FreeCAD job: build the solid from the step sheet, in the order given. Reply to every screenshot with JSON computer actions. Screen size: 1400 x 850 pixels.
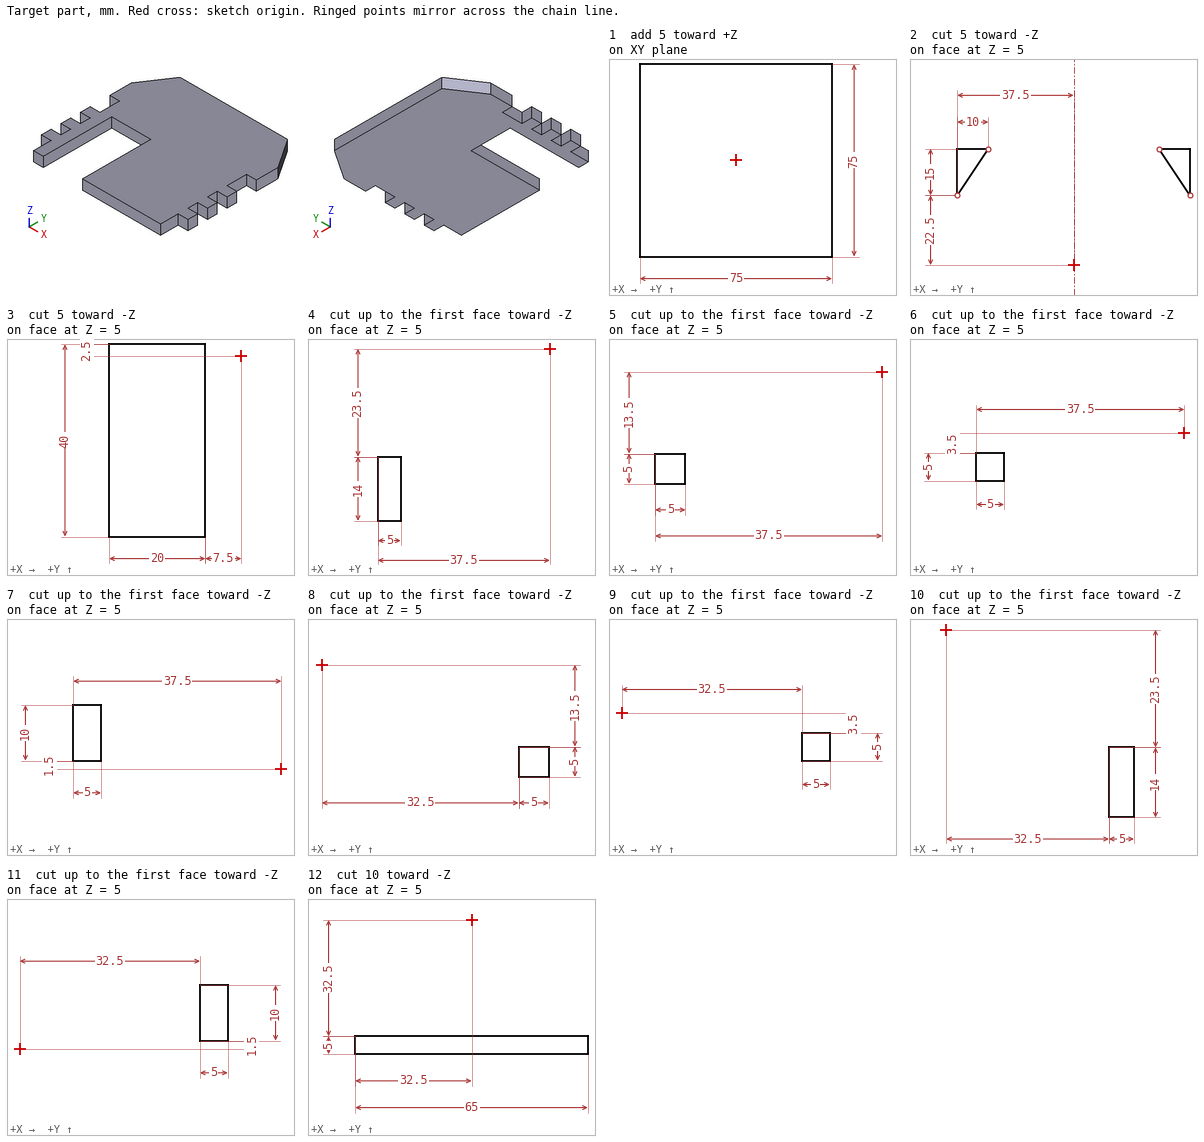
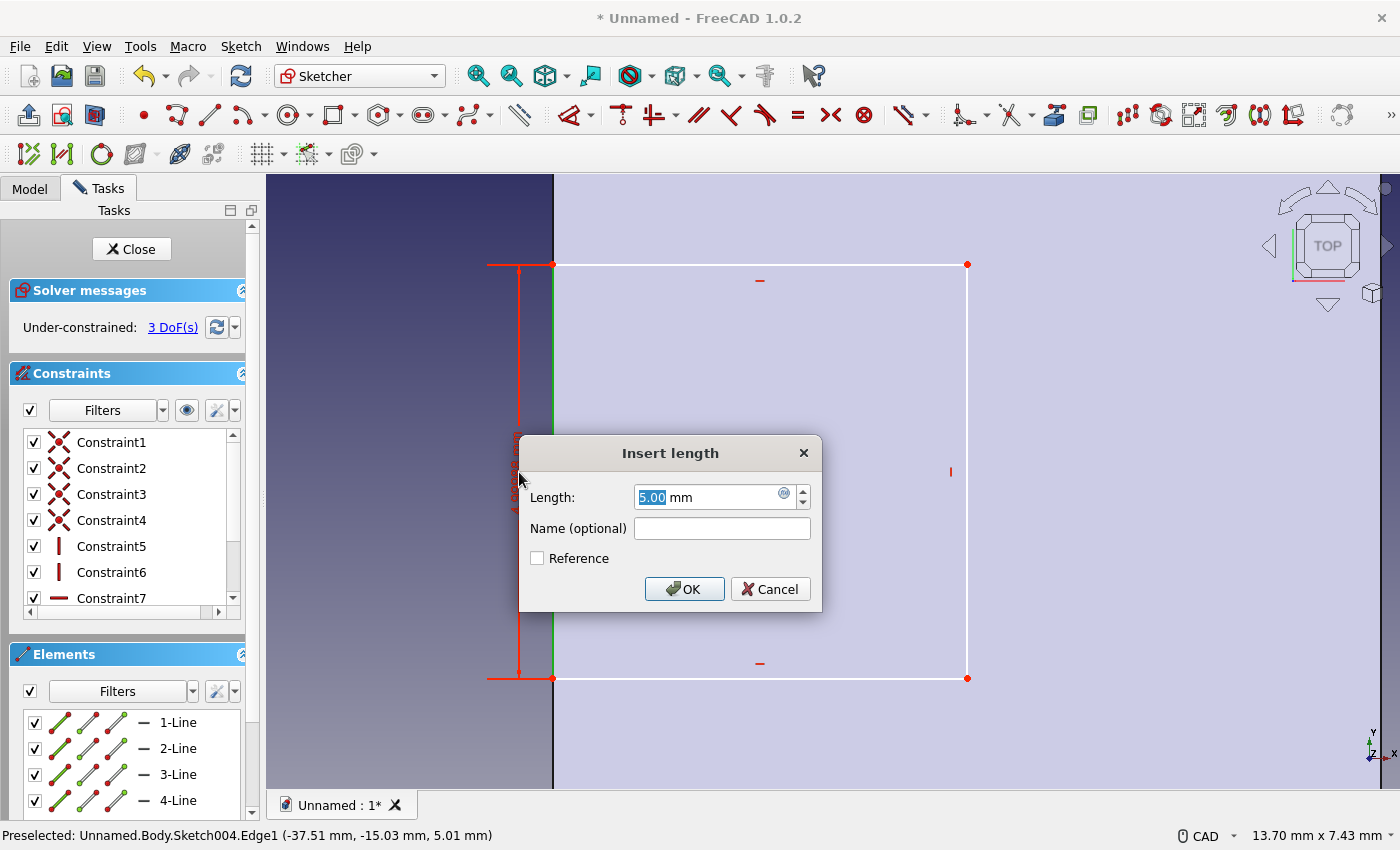
{"action": "type", "text": "5"}
{"action": "key", "text": "Return"}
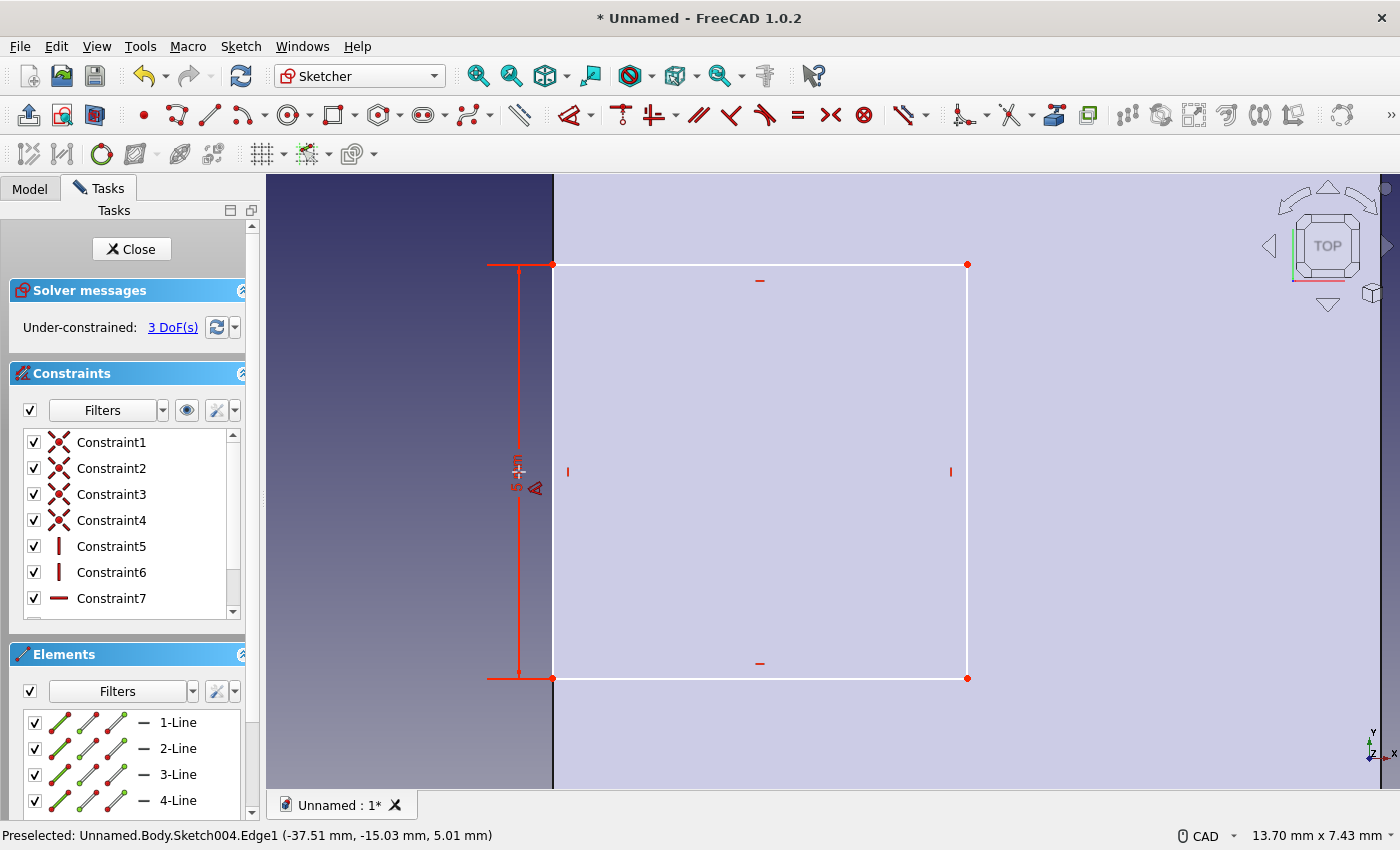
{"action": "left_click", "coordinate": [677, 679]}
{"action": "left_click", "coordinate": [760, 713]}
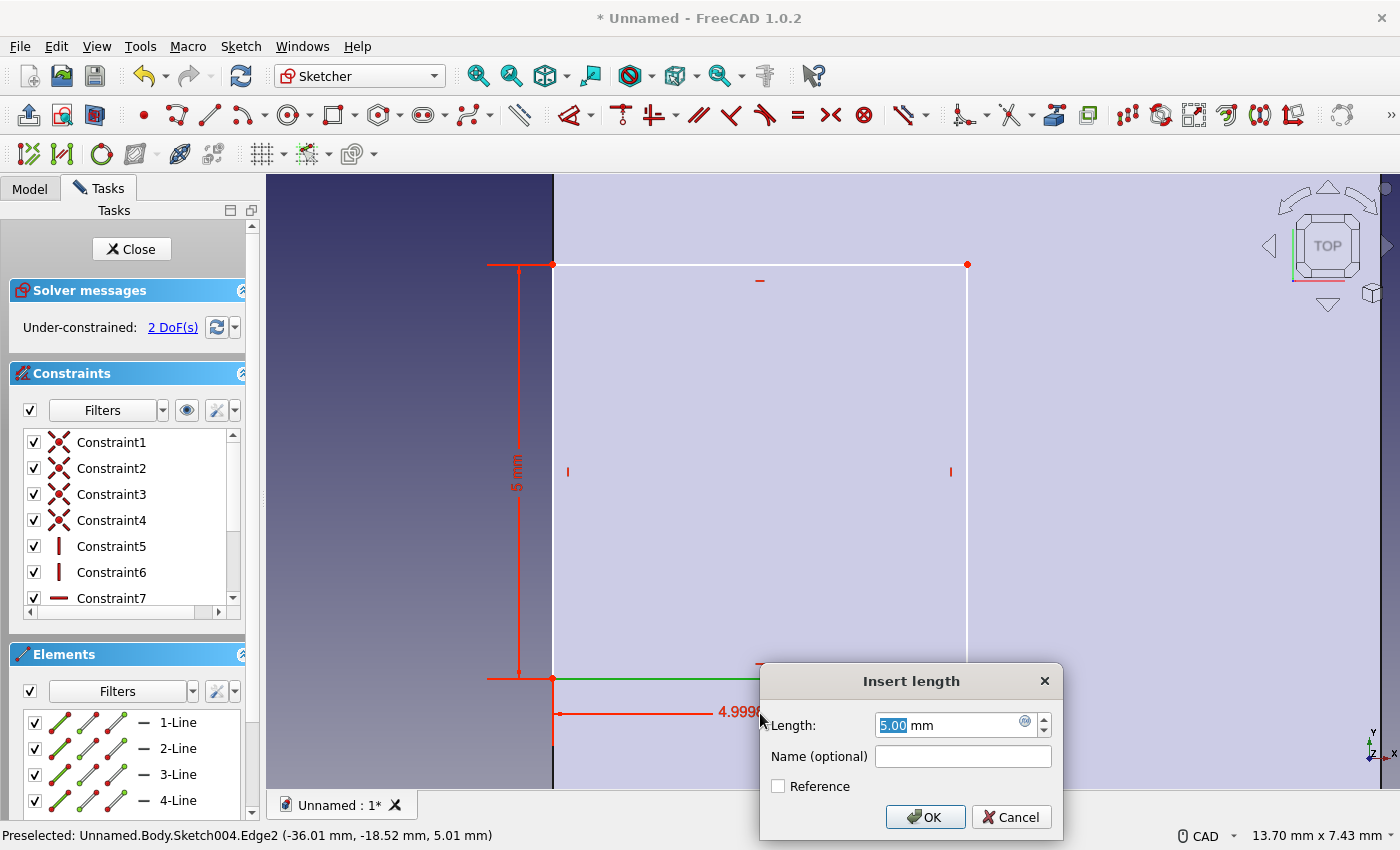
{"action": "type", "text": "5"}
{"action": "key", "text": "Return"}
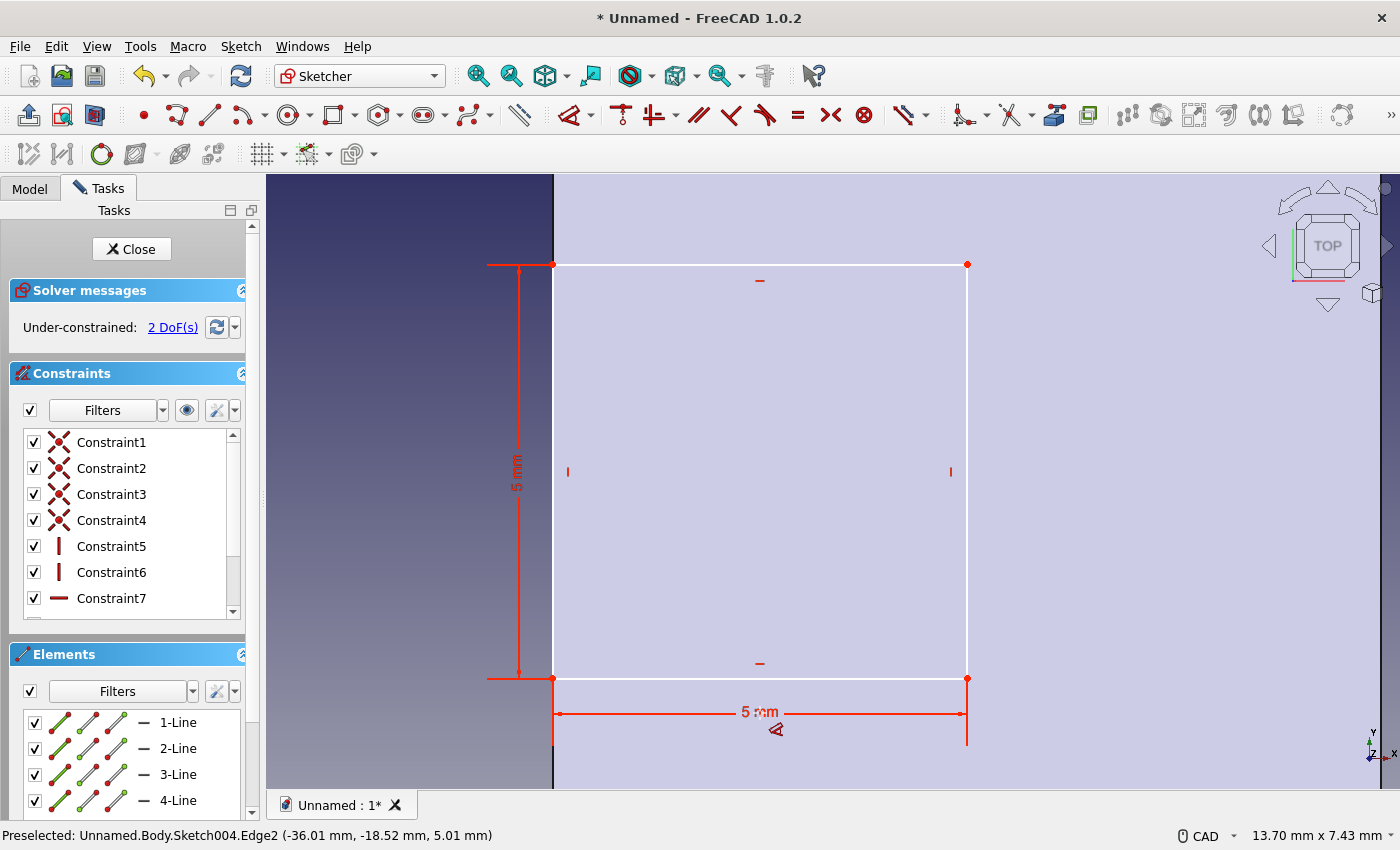
{"action": "left_click", "coordinate": [553, 265]}
{"action": "left_click", "coordinate": [894, 299]}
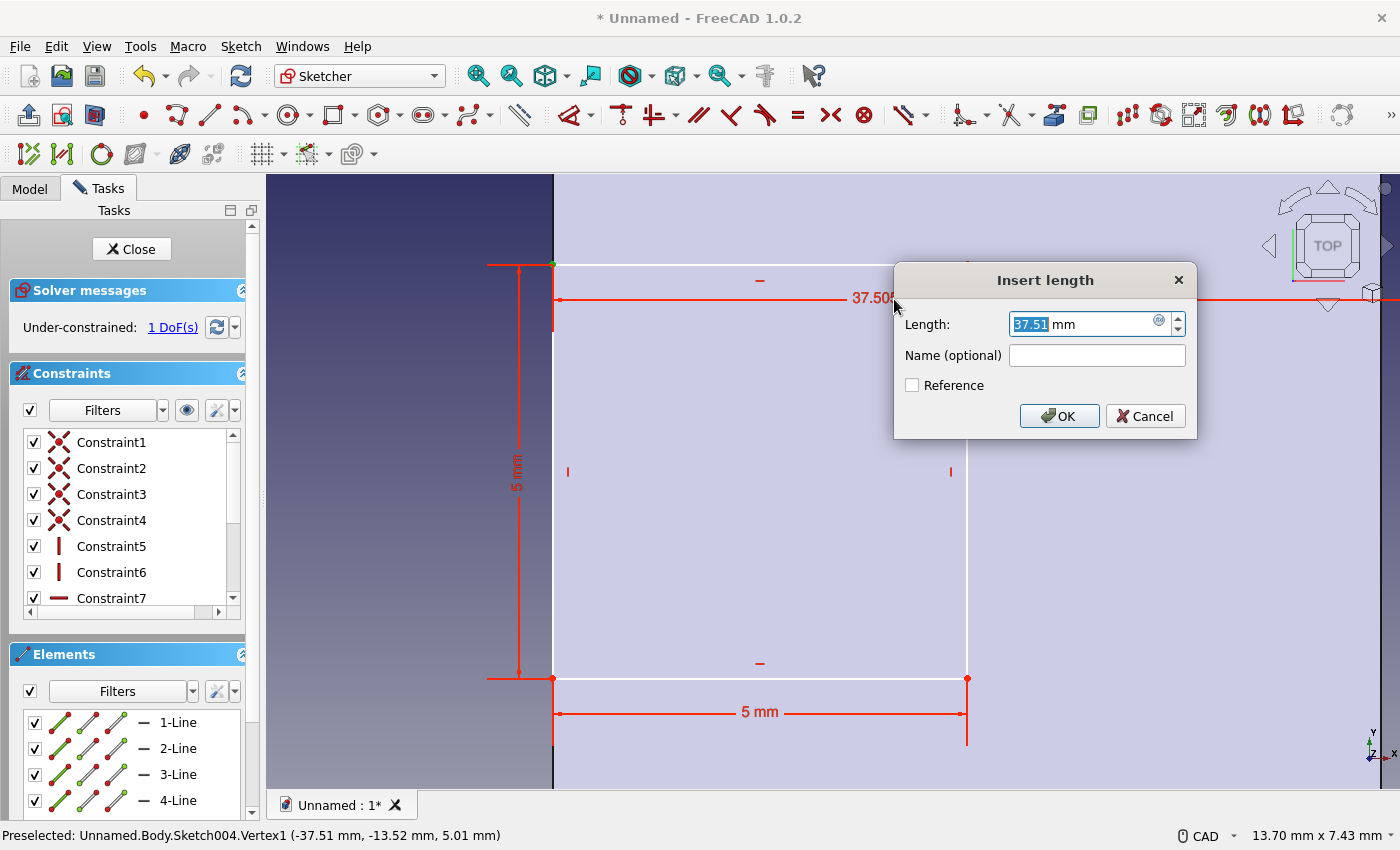
{"action": "type", "text": "37.5"}
{"action": "key", "text": "Return"}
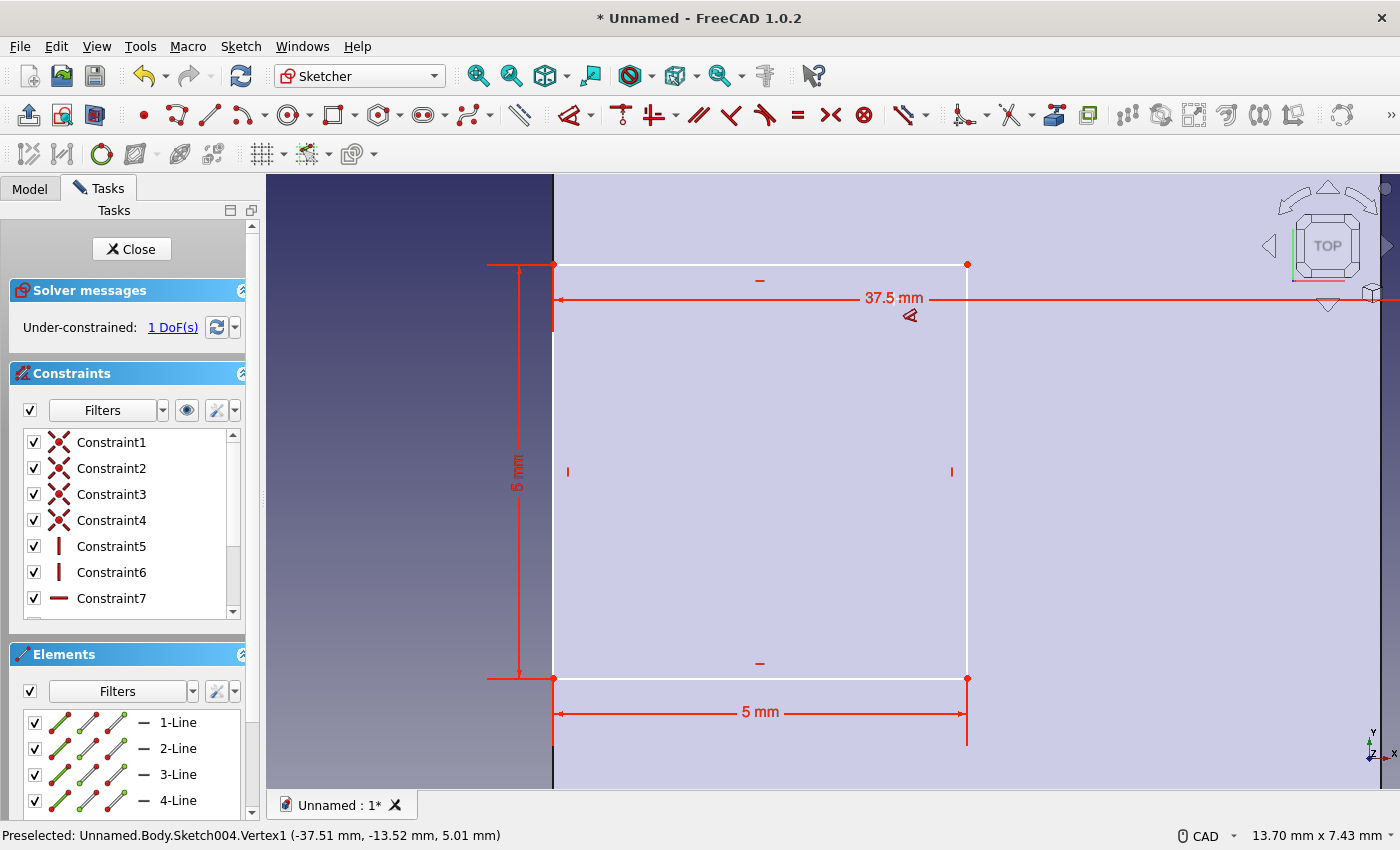
{"action": "left_click", "coordinate": [553, 265]}
{"action": "left_click", "coordinate": [519, 233]}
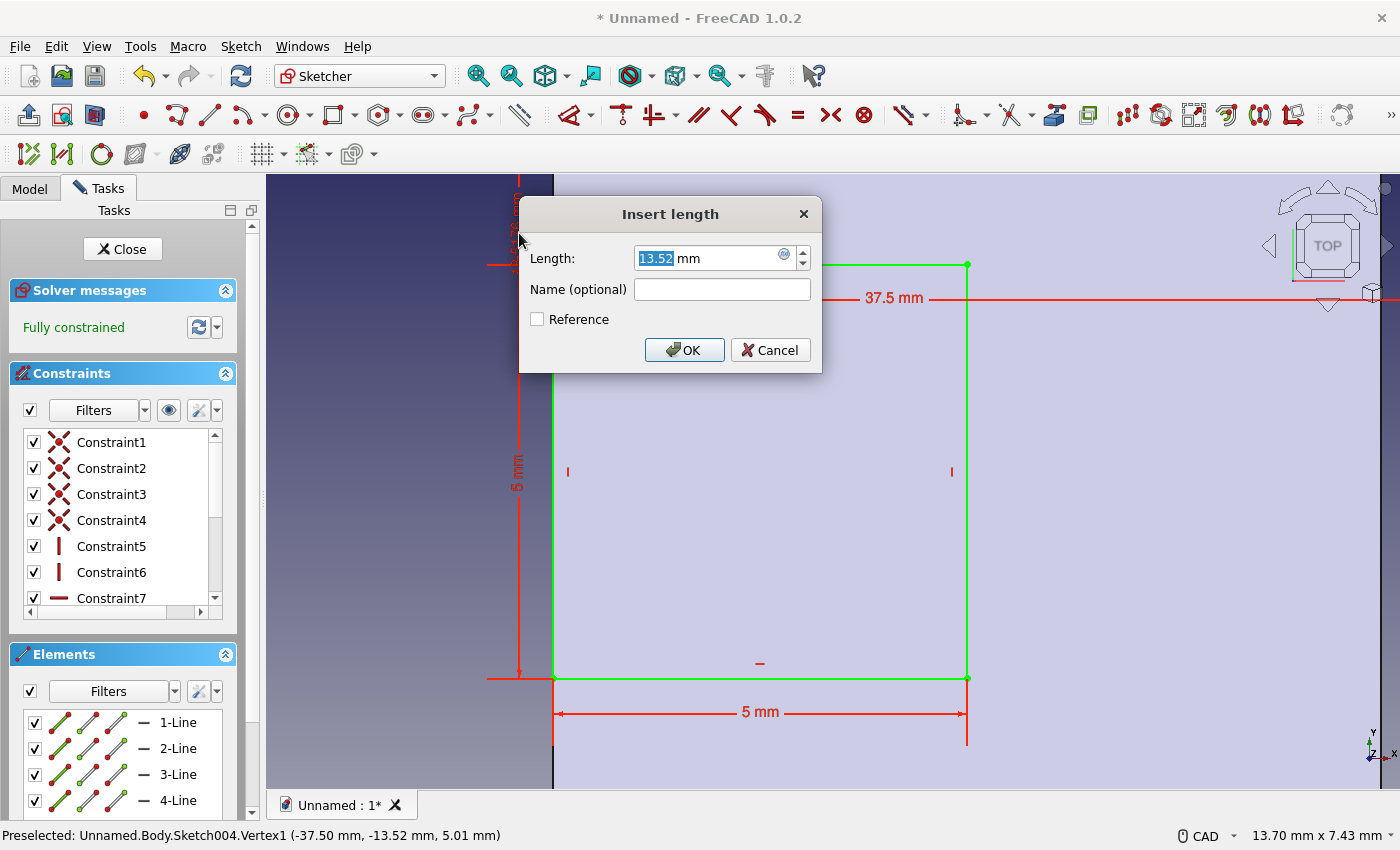
{"action": "type", "text": "13.5"}
{"action": "key", "text": "Return"}
{"action": "key", "text": "Escape"}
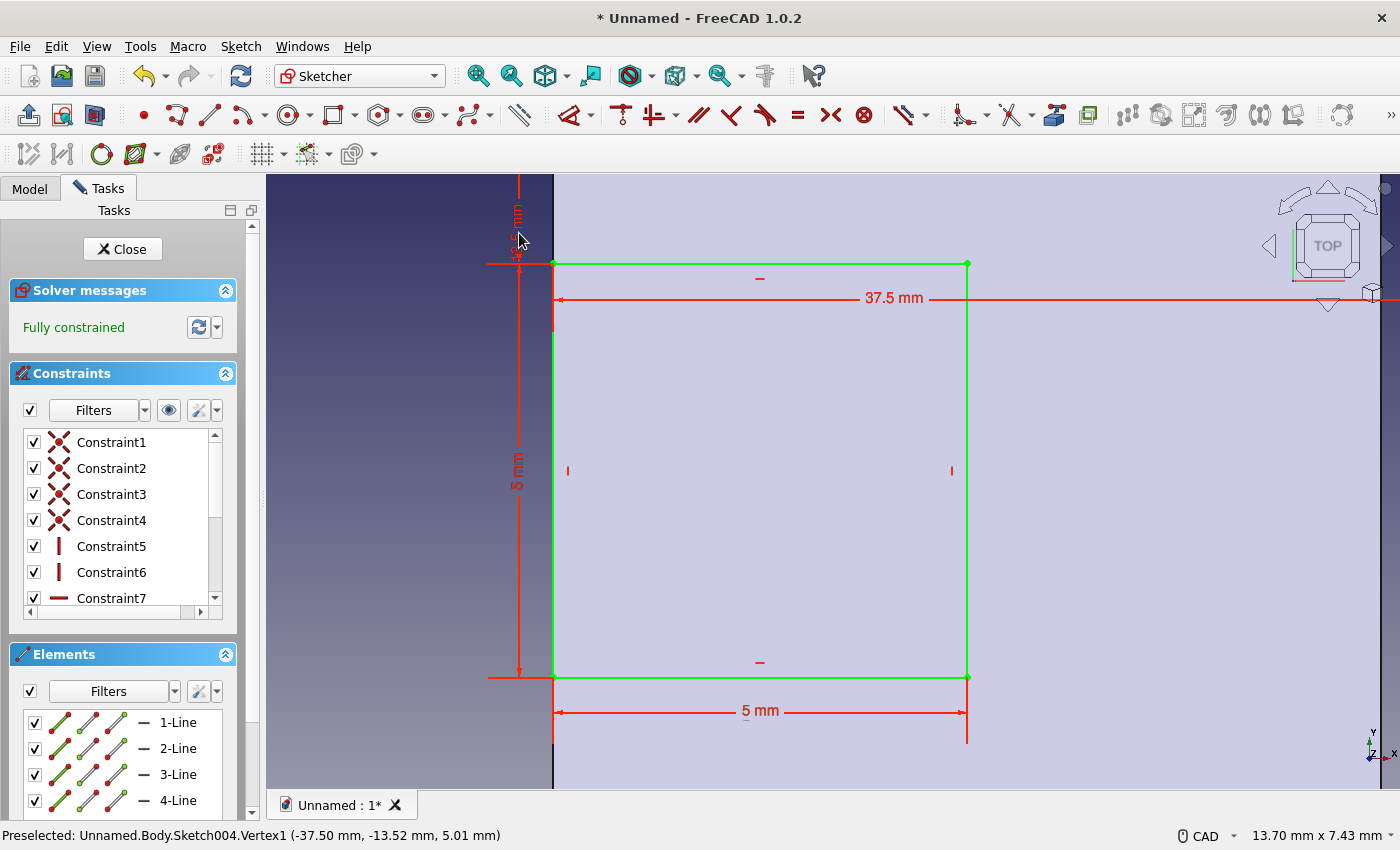
{"action": "left_click", "coordinate": [123, 249]}